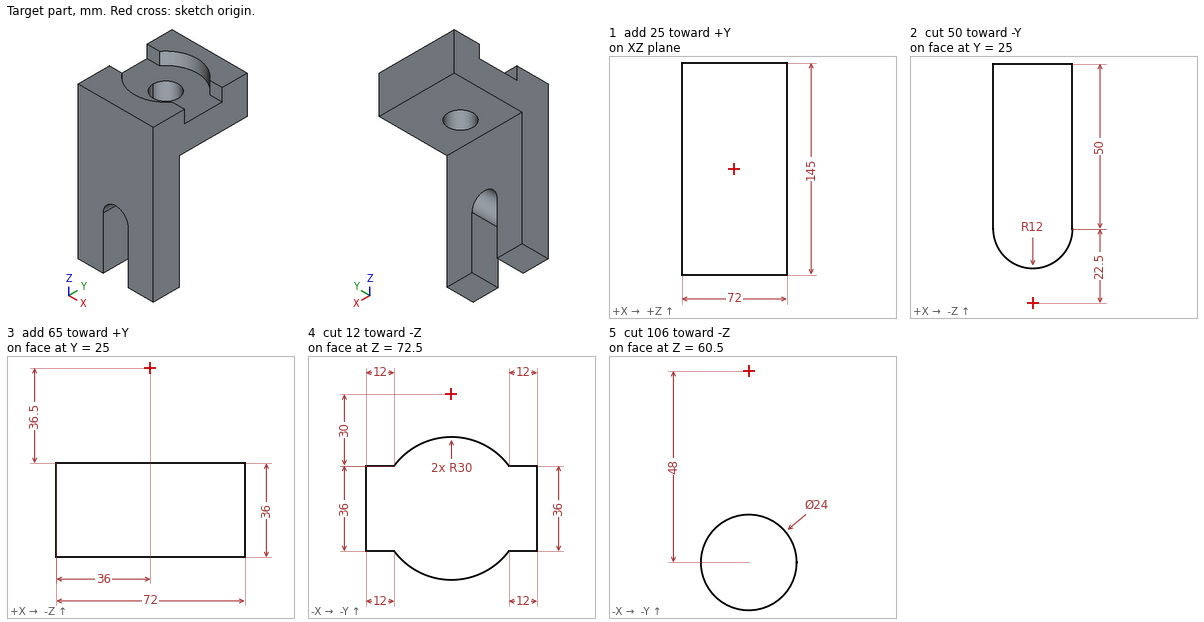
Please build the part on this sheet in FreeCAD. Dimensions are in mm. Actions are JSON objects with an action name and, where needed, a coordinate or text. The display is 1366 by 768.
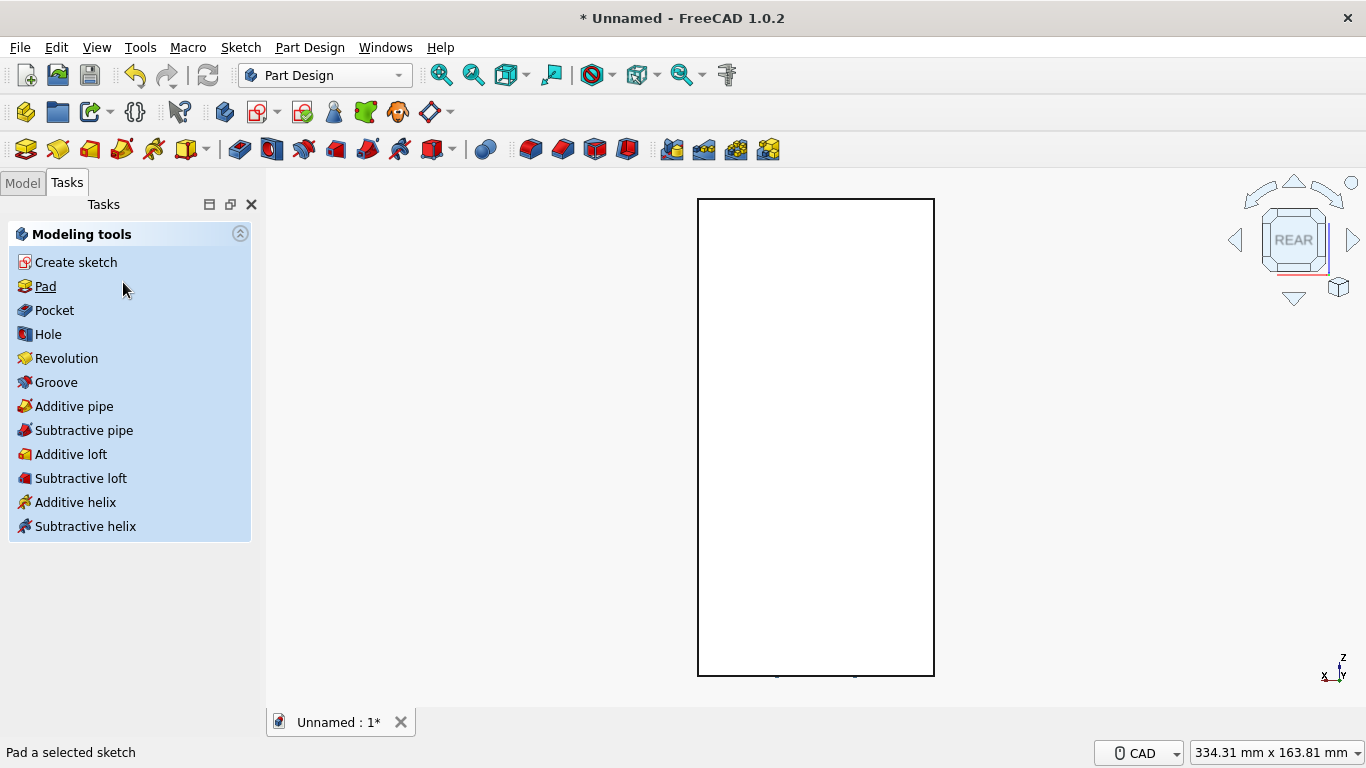
{"action": "left_click", "coordinate": [240, 150]}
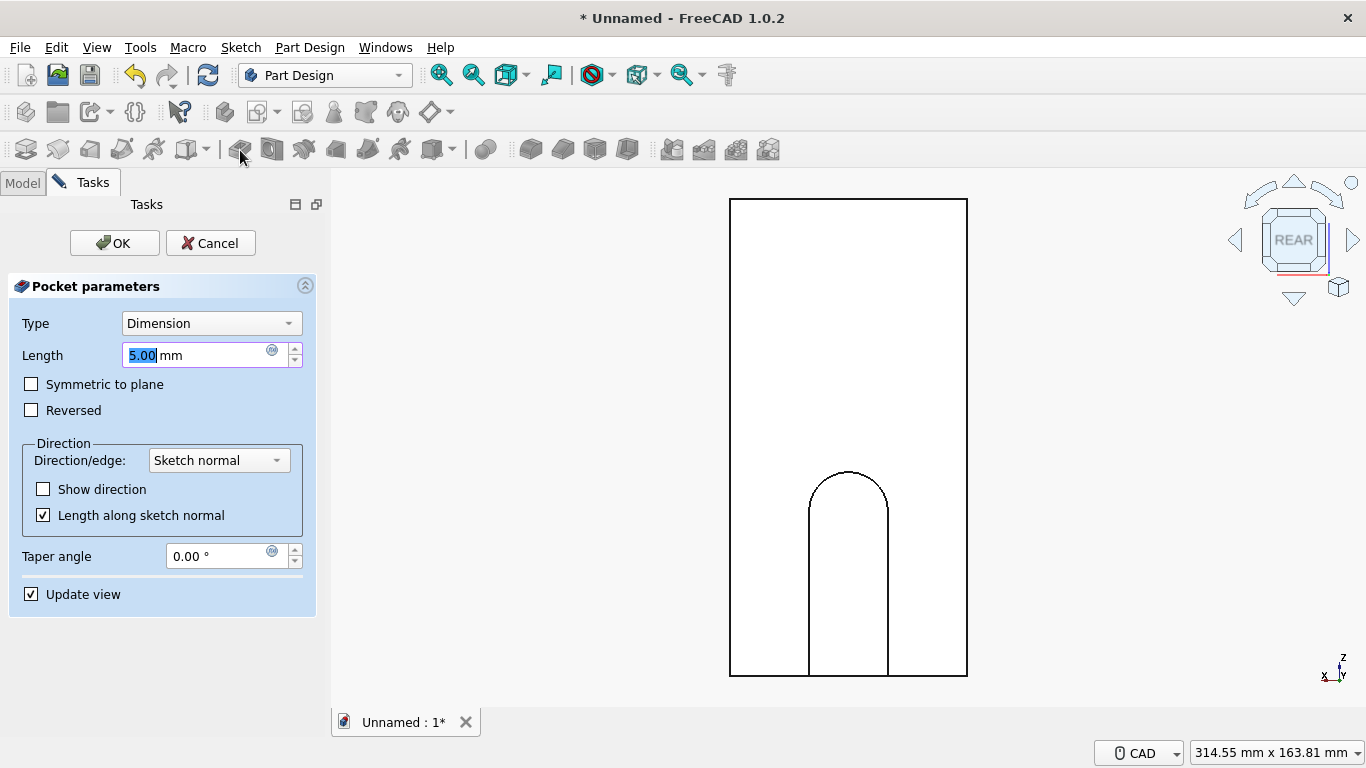
{"action": "type", "text": "50"}
{"action": "key", "text": "Tab"}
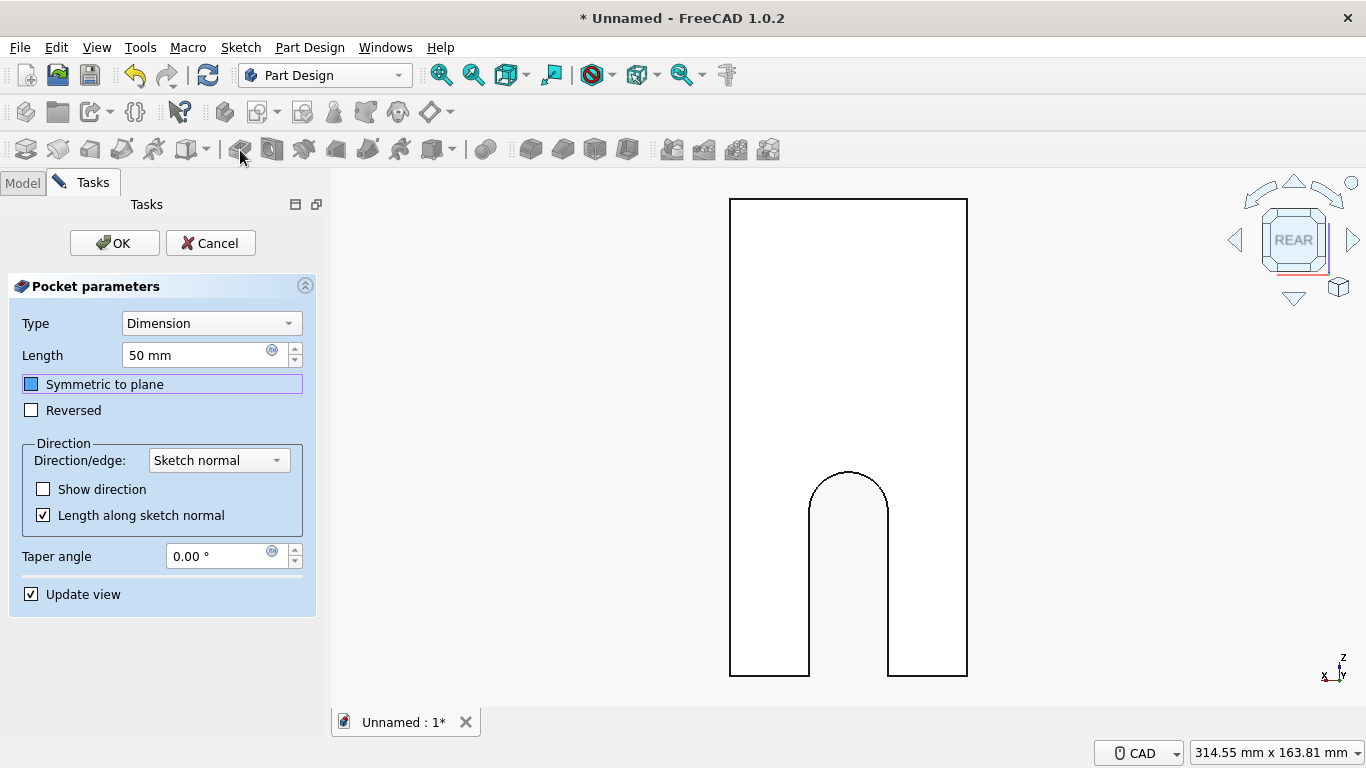
{"action": "left_click", "coordinate": [115, 243]}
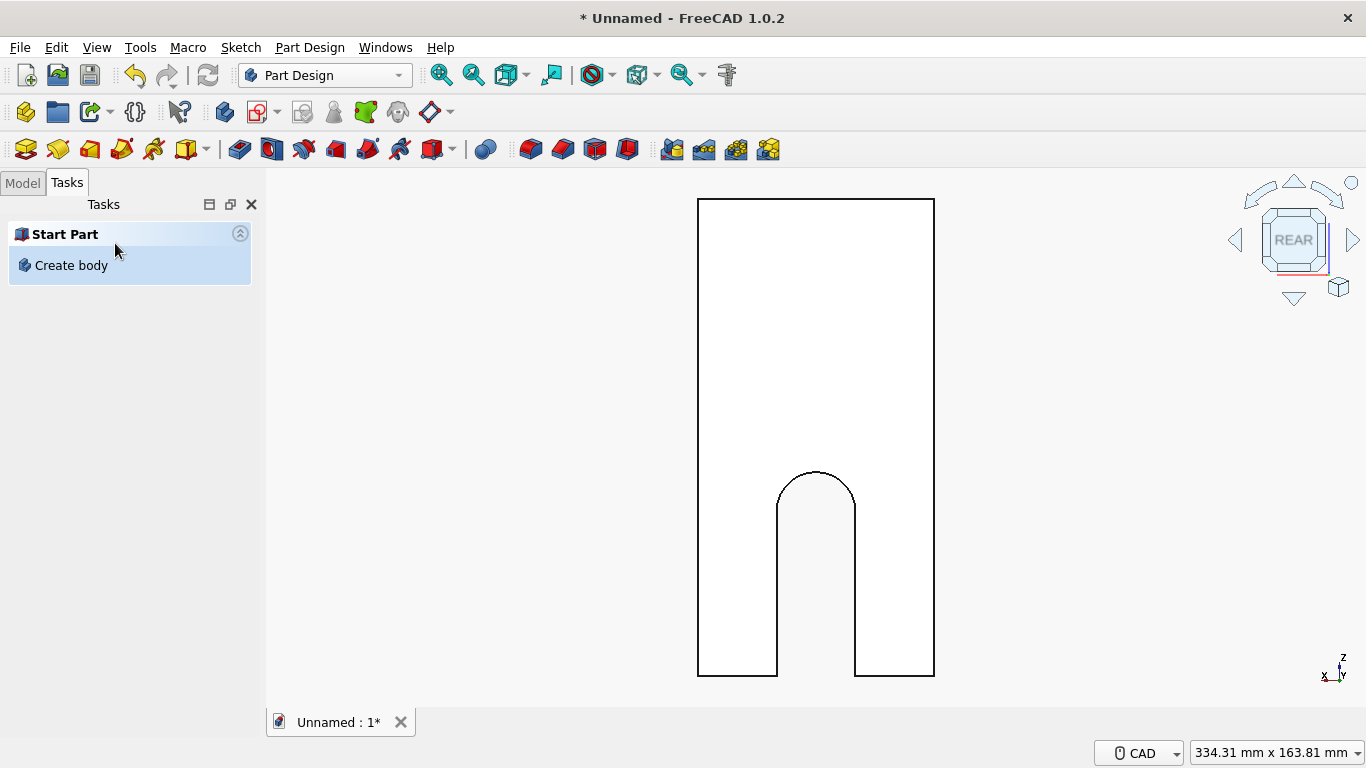
{"action": "left_click", "coordinate": [816, 368]}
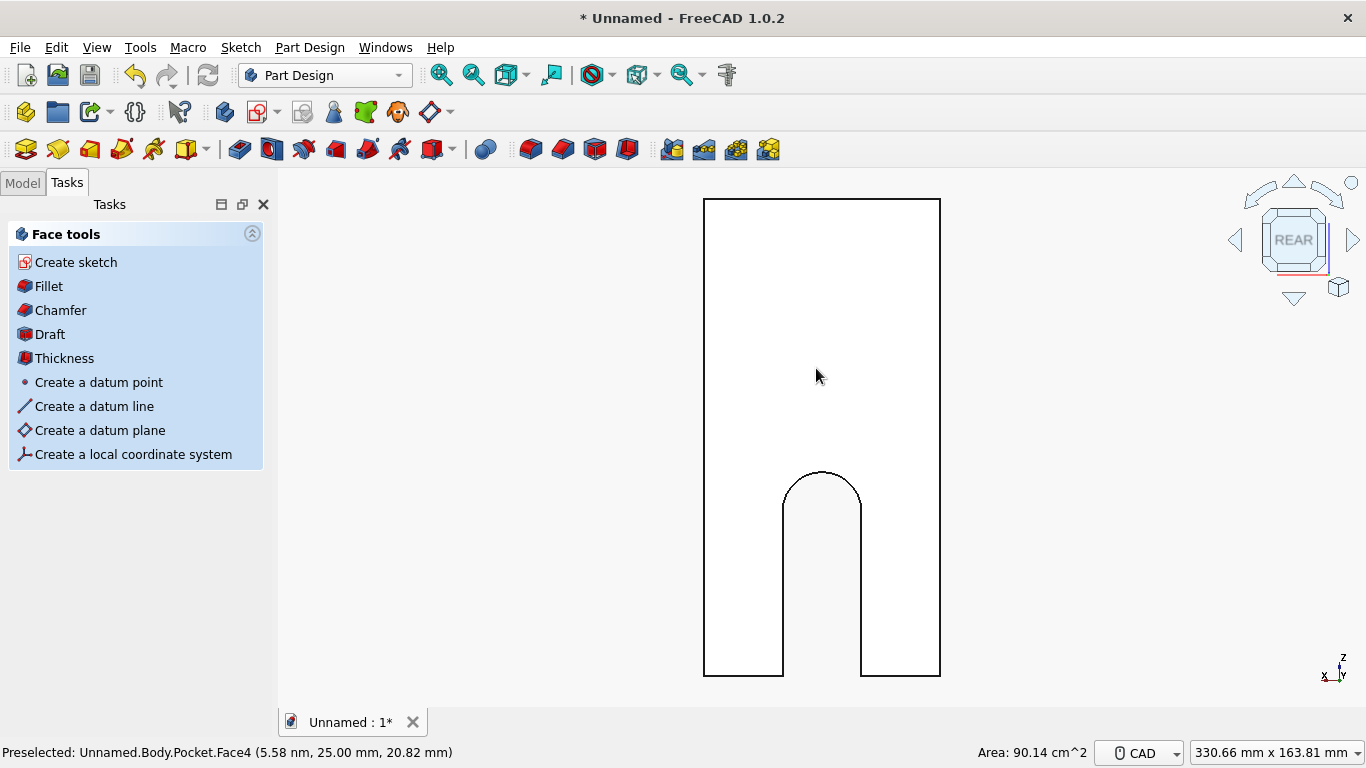
{"action": "left_click", "coordinate": [258, 112]}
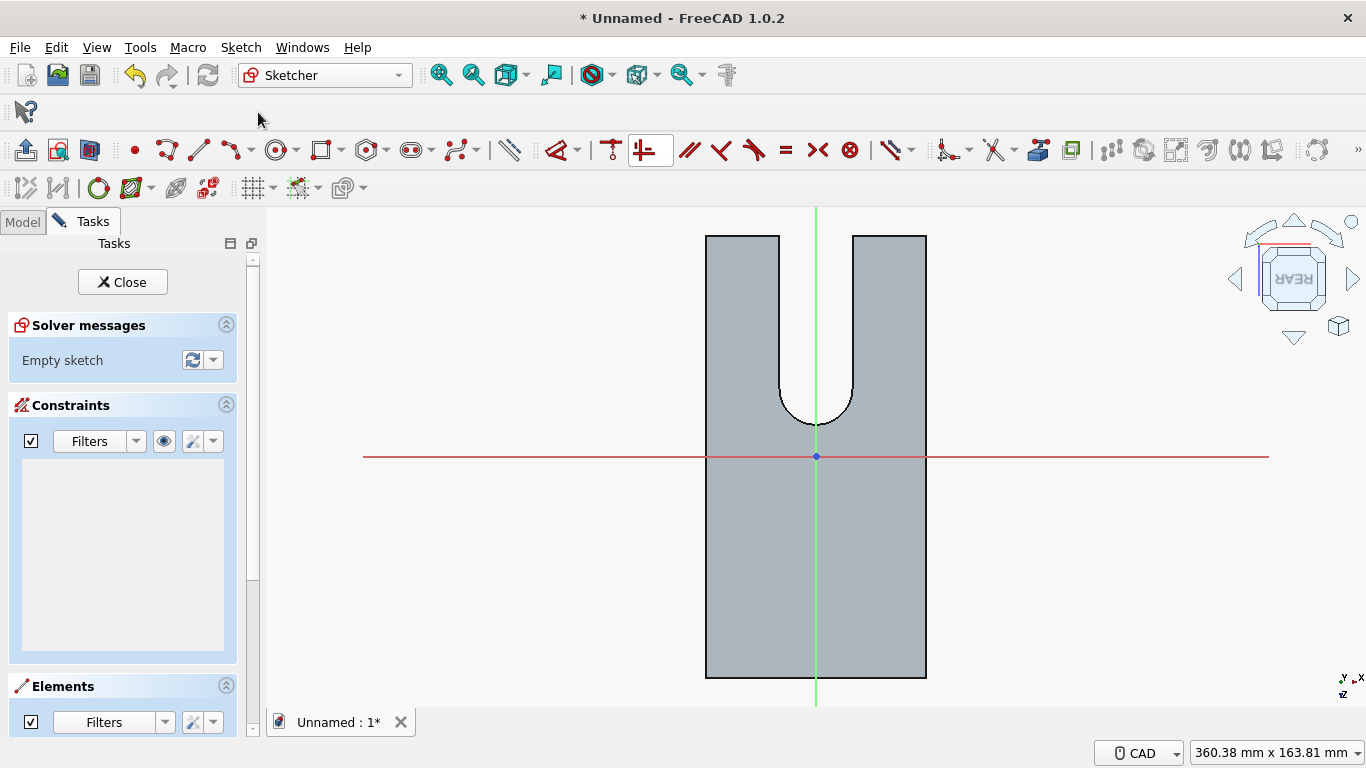
{"action": "scroll", "coordinate": [438, 235], "scroll_direction": "down", "scroll_amount": 1}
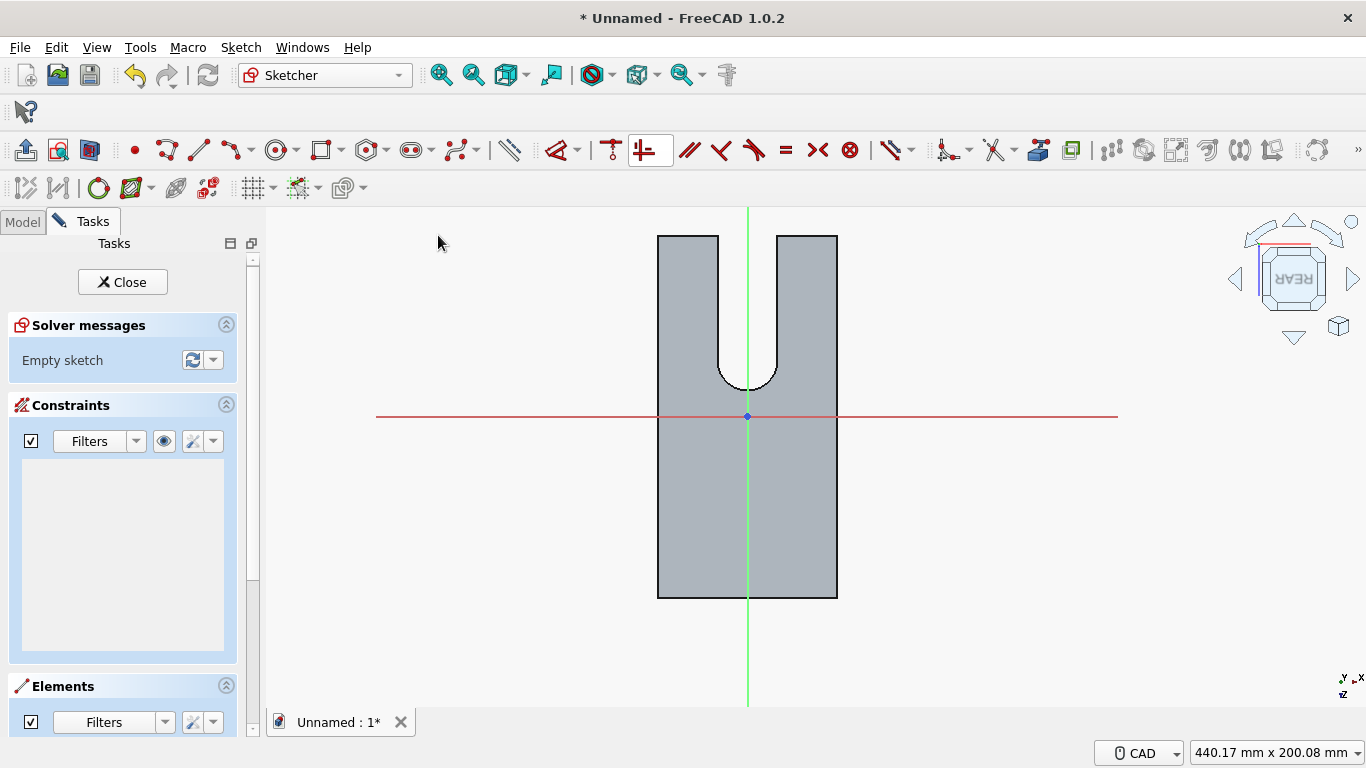
{"action": "scroll", "coordinate": [748, 569], "scroll_direction": "up", "scroll_amount": 3}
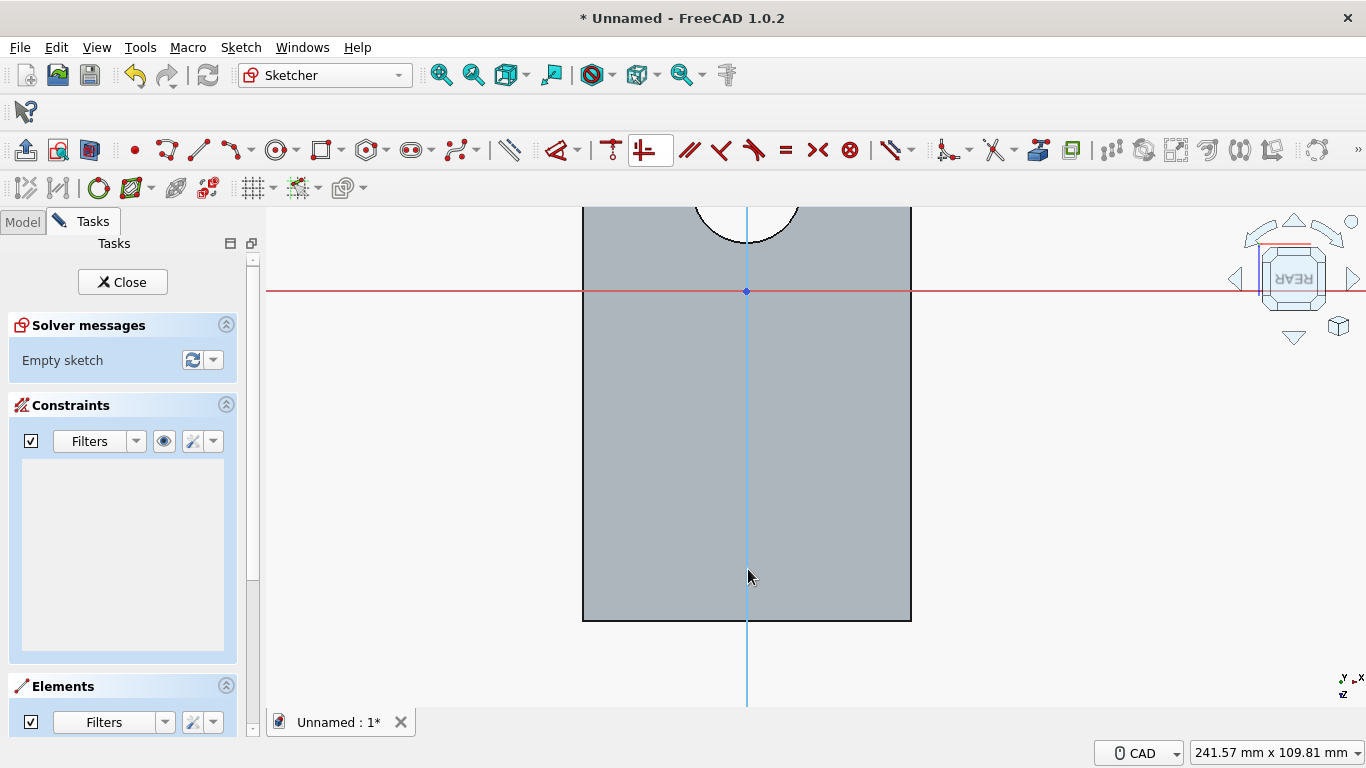
{"action": "left_click", "coordinate": [322, 150]}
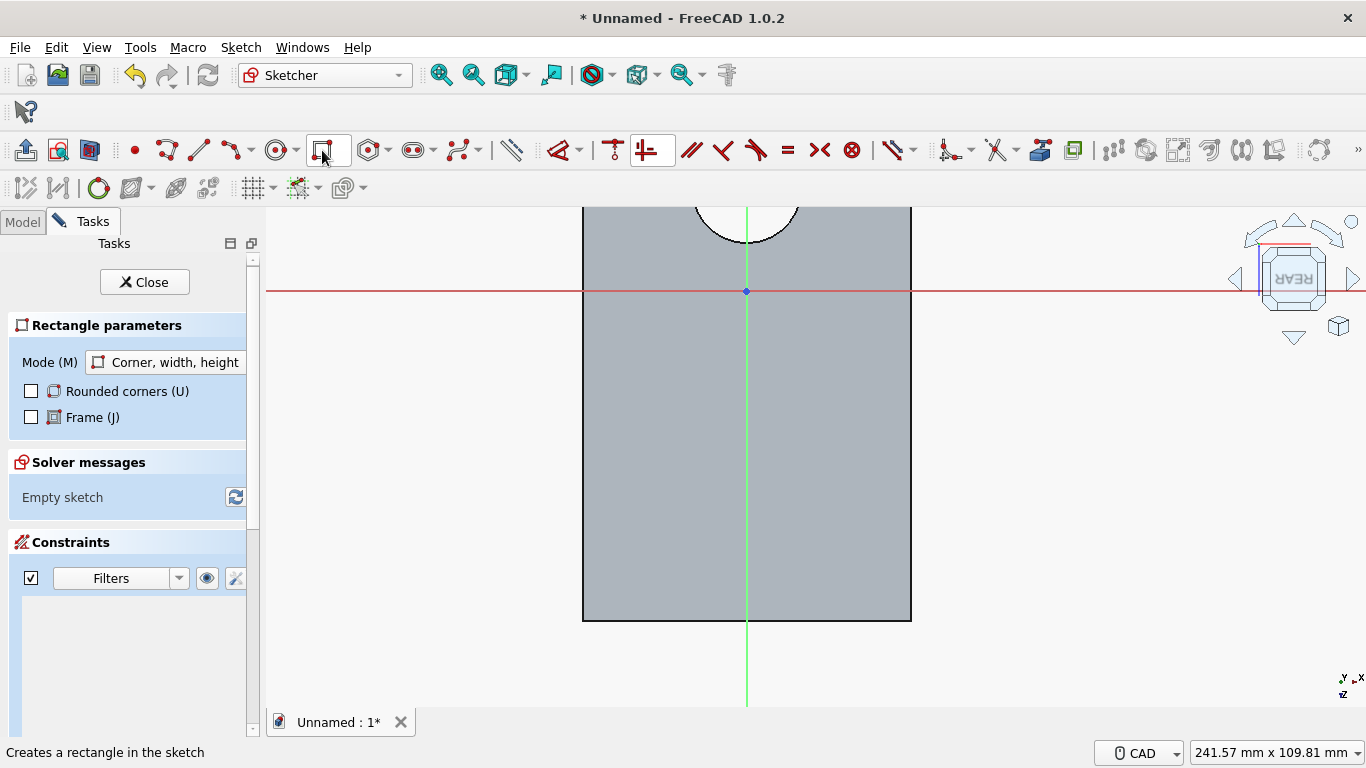
{"action": "left_click", "coordinate": [583, 457]}
{"action": "mouse_move", "coordinate": [911, 621]}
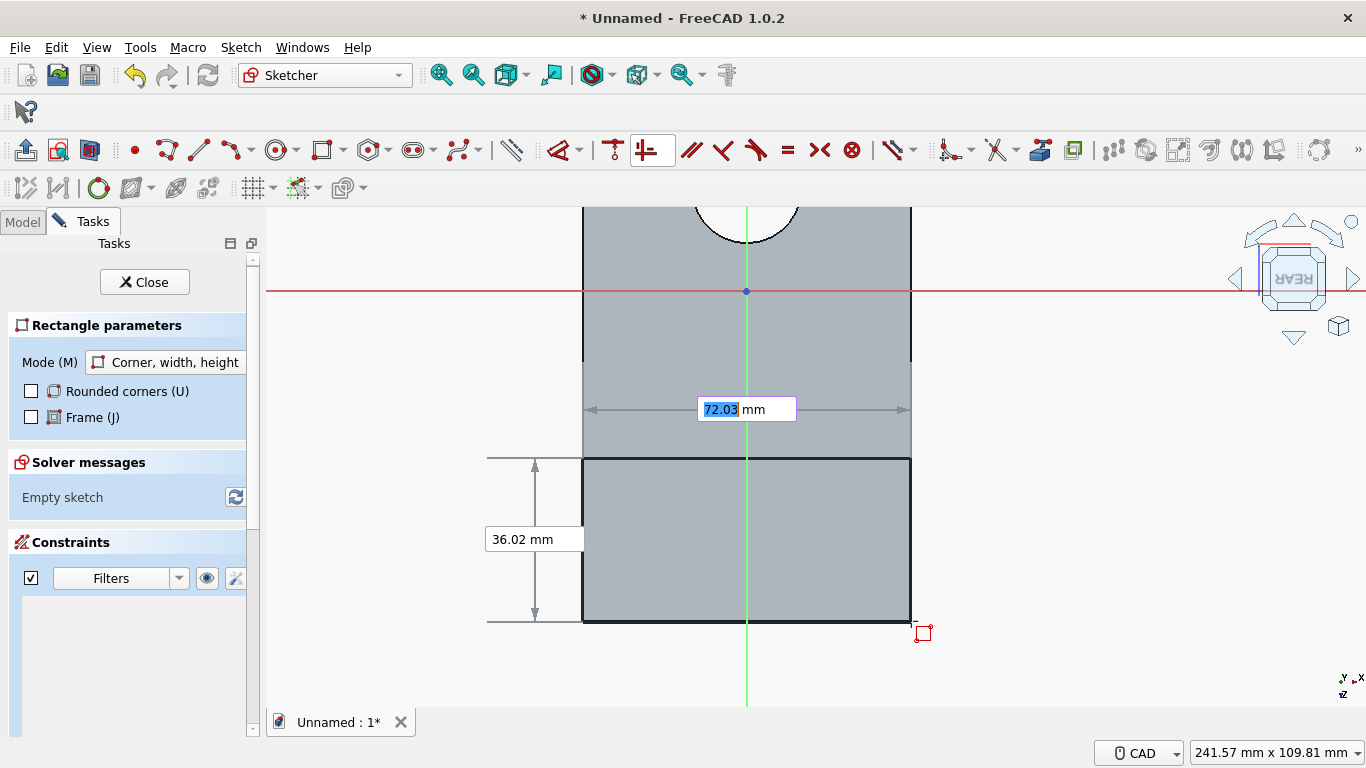
{"action": "type", "text": "72"}
{"action": "key", "text": "Tab"}
{"action": "type", "text": "36"}
{"action": "key", "text": "Return"}
{"action": "key", "text": "Escape"}